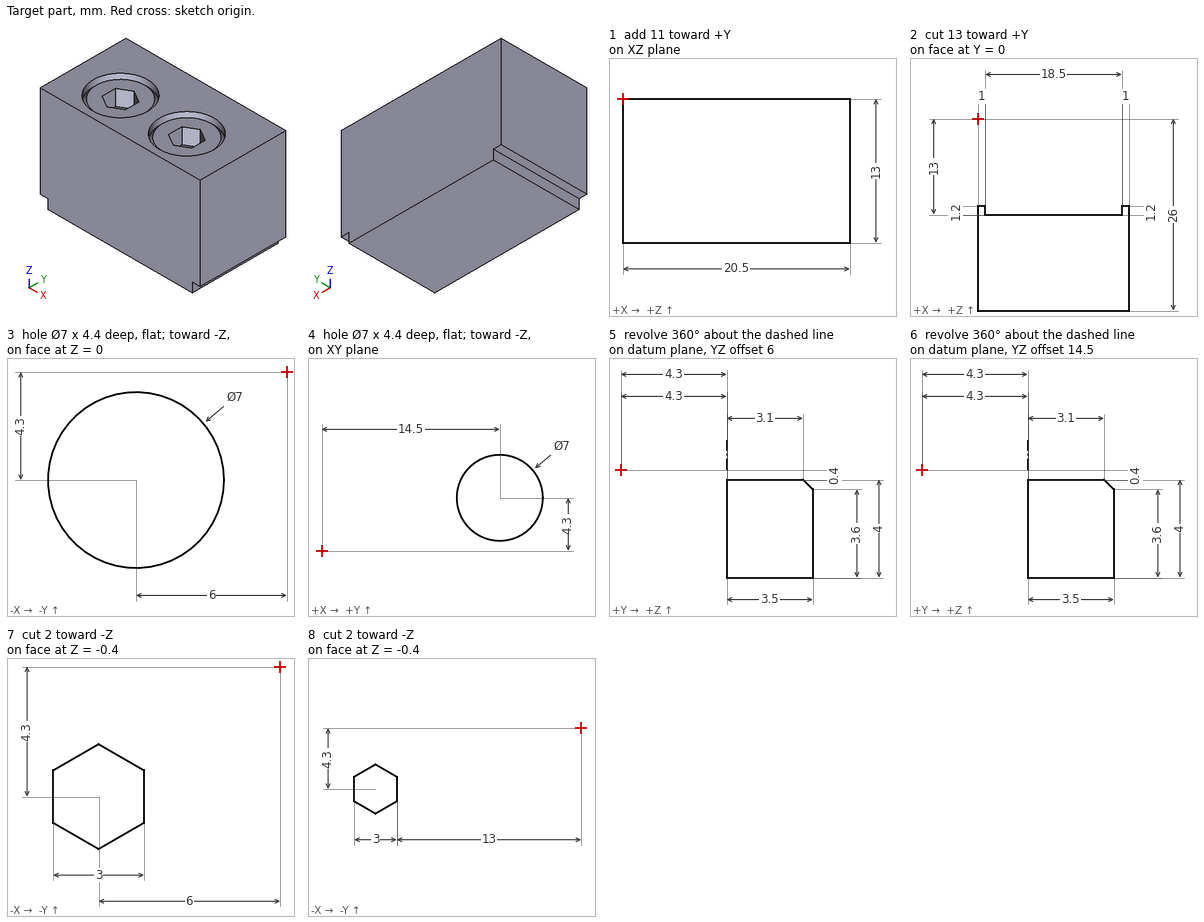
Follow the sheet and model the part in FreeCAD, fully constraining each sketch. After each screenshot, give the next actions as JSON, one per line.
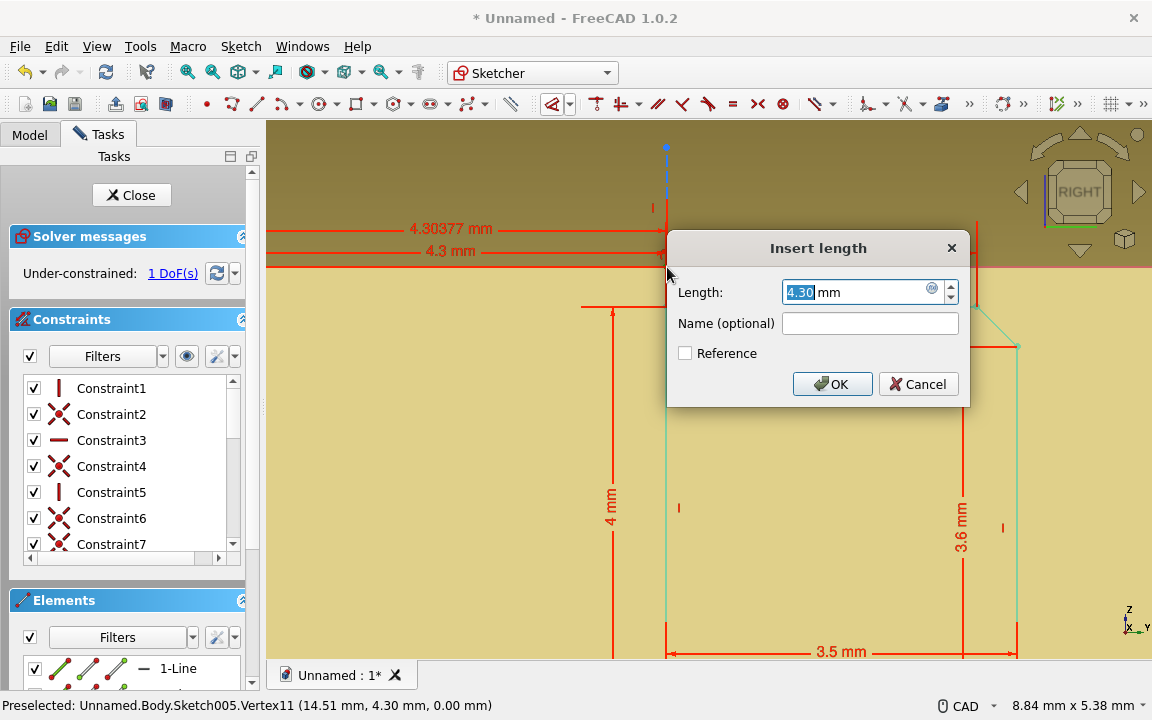
{"action": "type", "text": "4.3"}
{"action": "key", "text": "Return"}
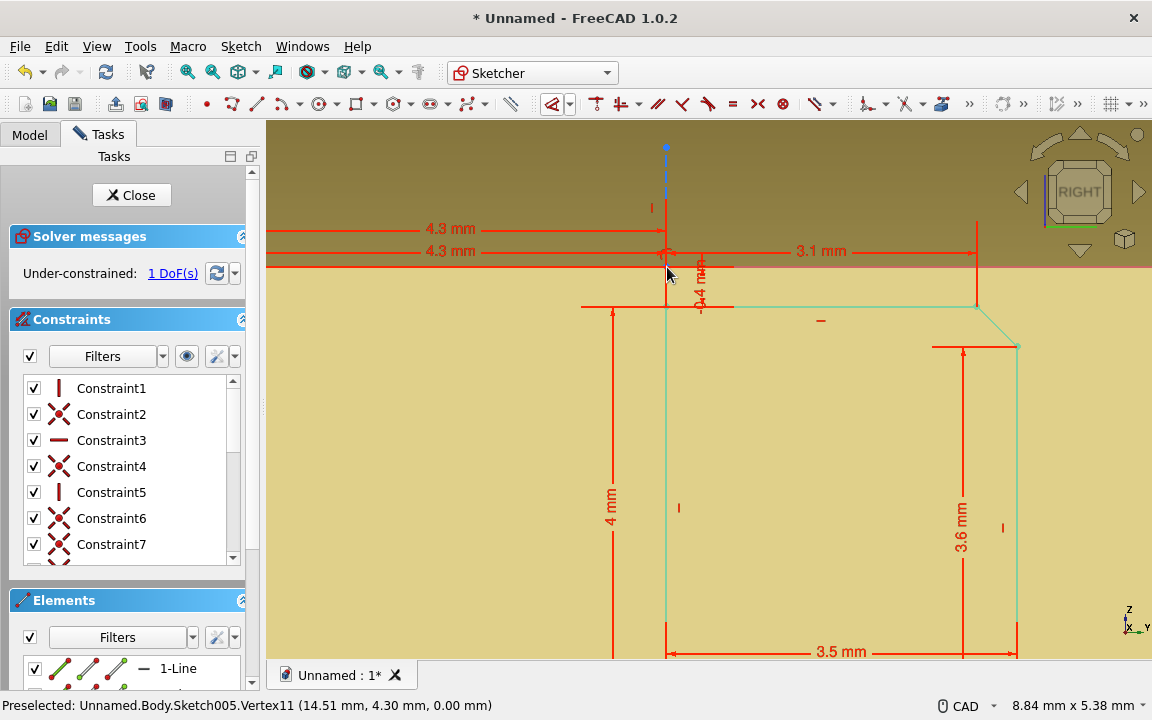
{"action": "left_click", "coordinate": [132, 195]}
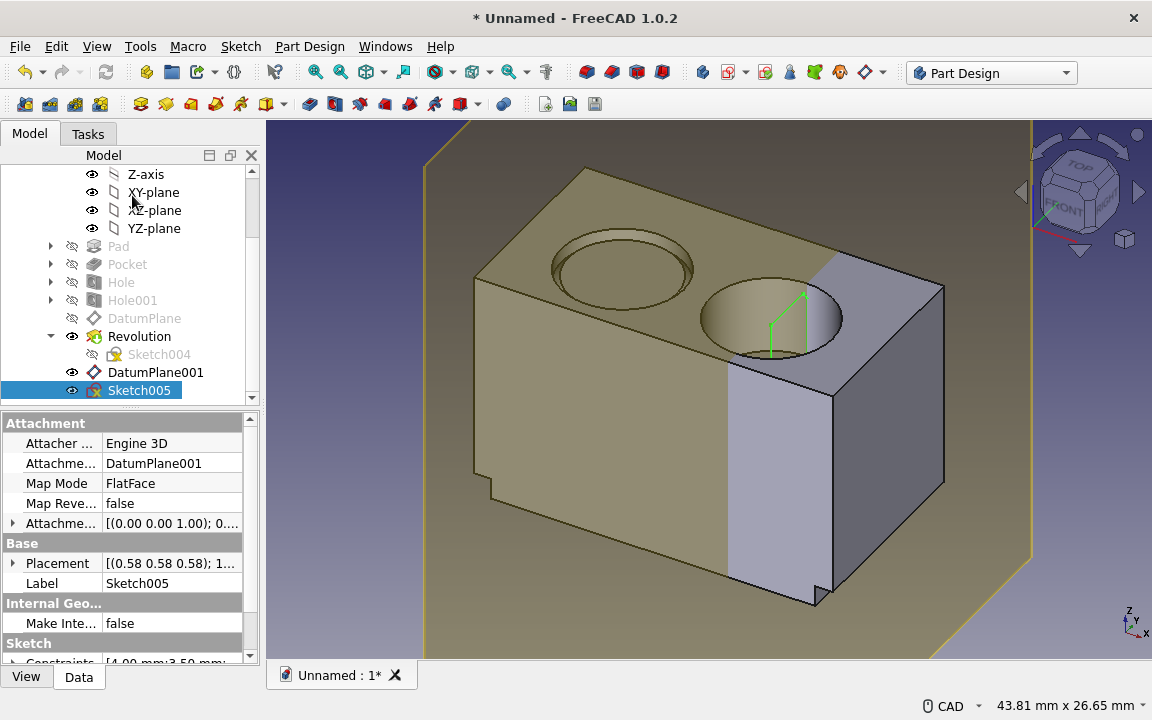
{"action": "left_click", "coordinate": [166, 104]}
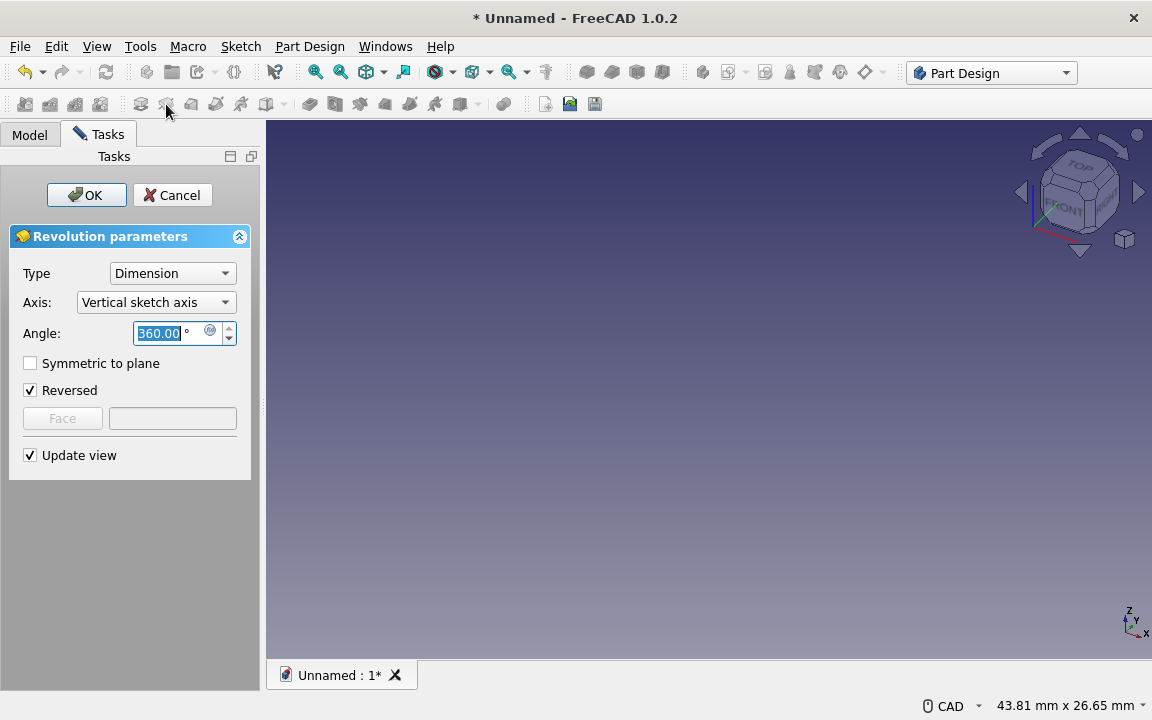
{"action": "left_click", "coordinate": [157, 302]}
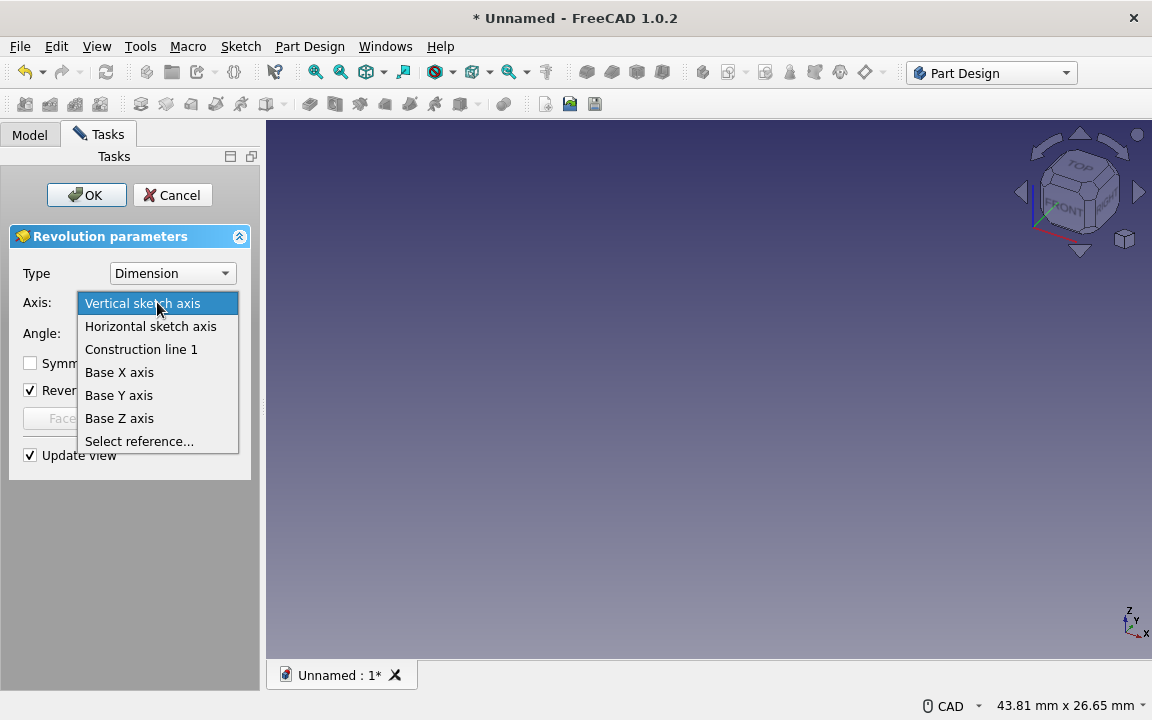
{"action": "left_click", "coordinate": [156, 350]}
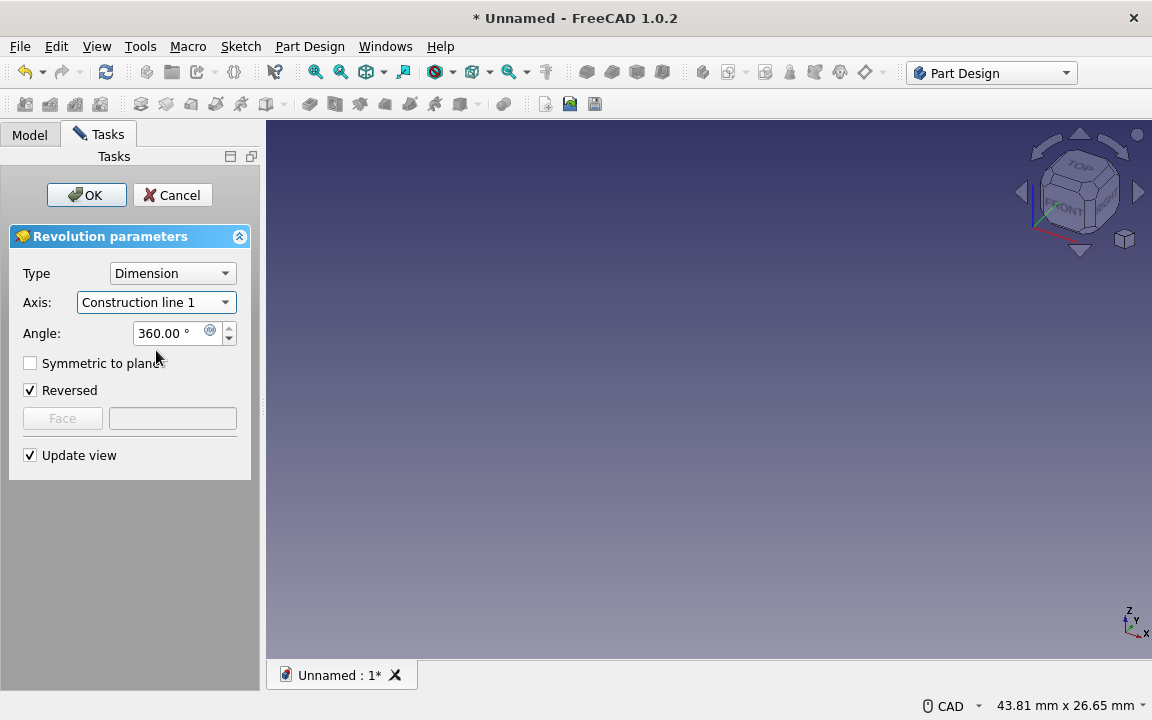
{"action": "left_click", "coordinate": [87, 195]}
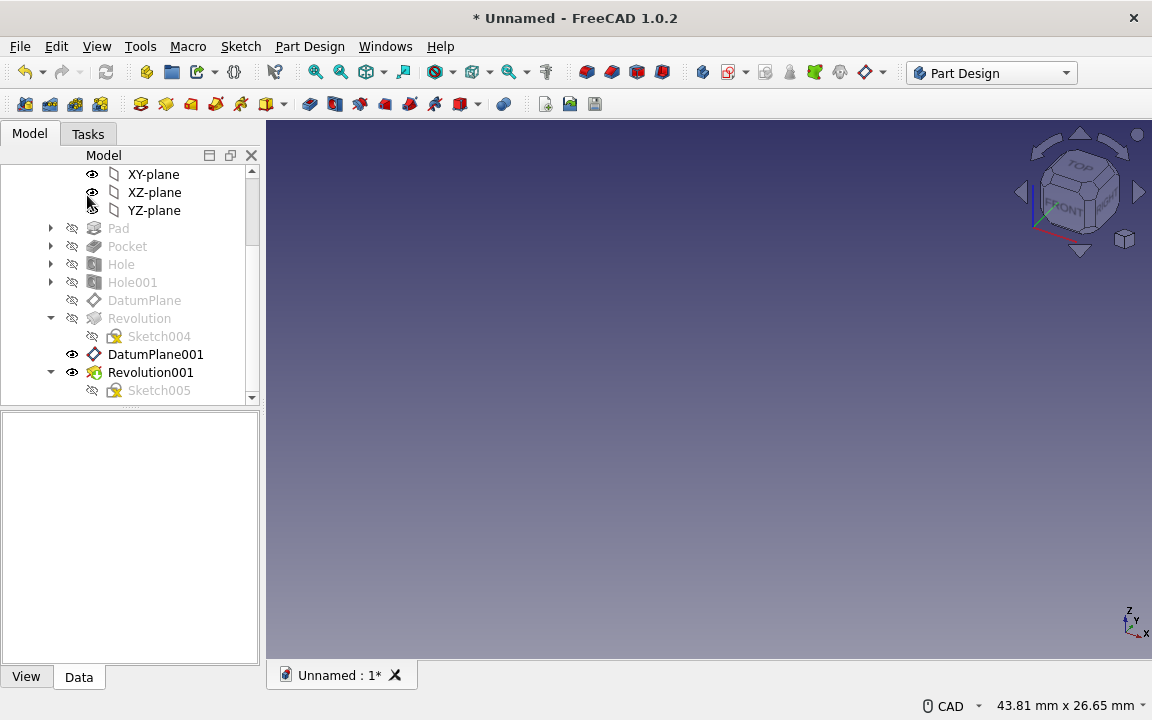
{"action": "left_click", "coordinate": [117, 354]}
{"action": "key", "text": "space"}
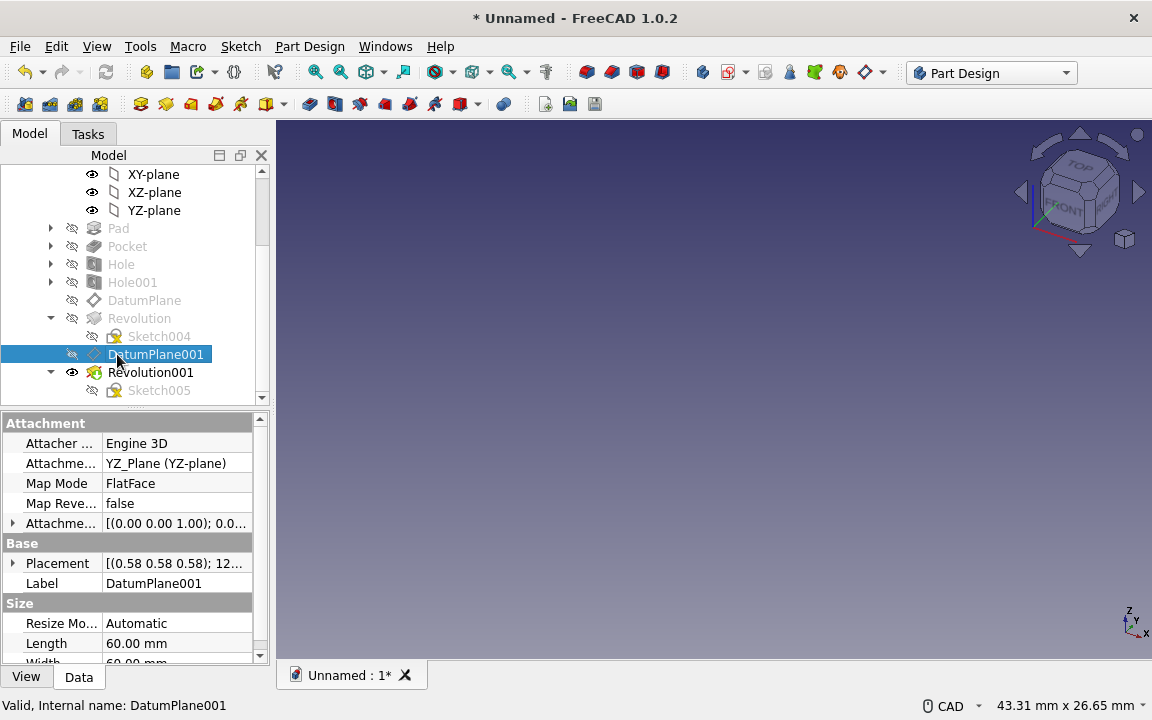
{"action": "left_click", "coordinate": [316, 72]}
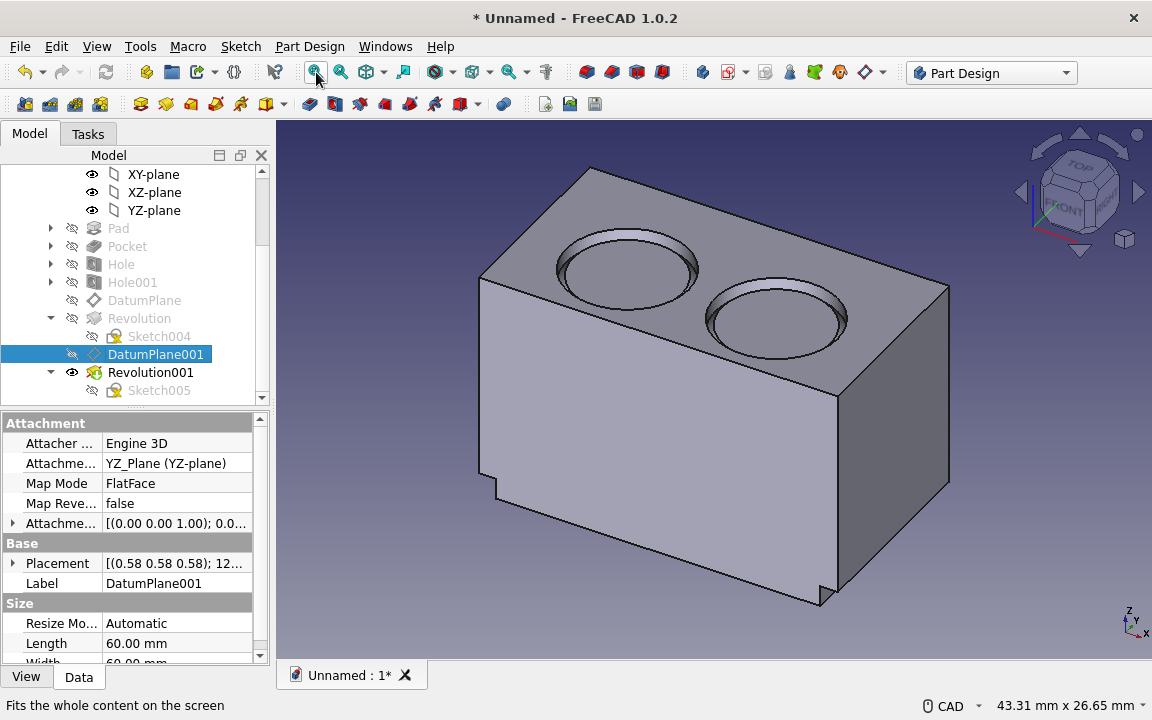
{"action": "left_click", "coordinate": [627, 275]}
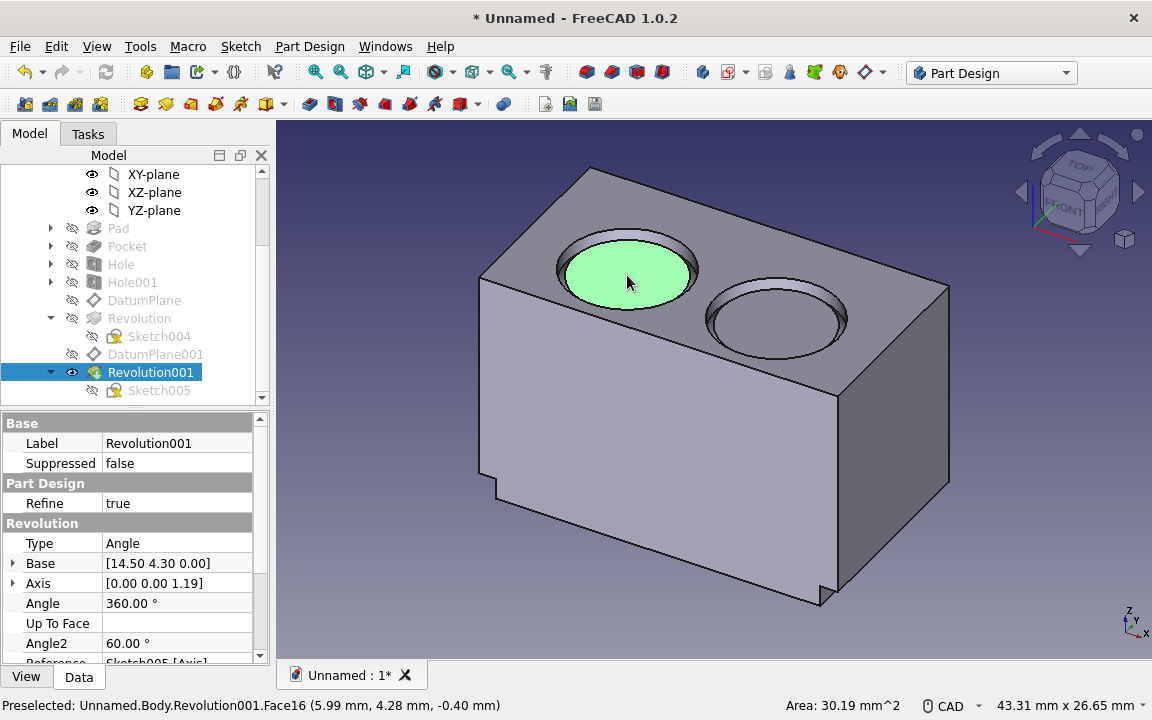
{"action": "left_click", "coordinate": [728, 72]}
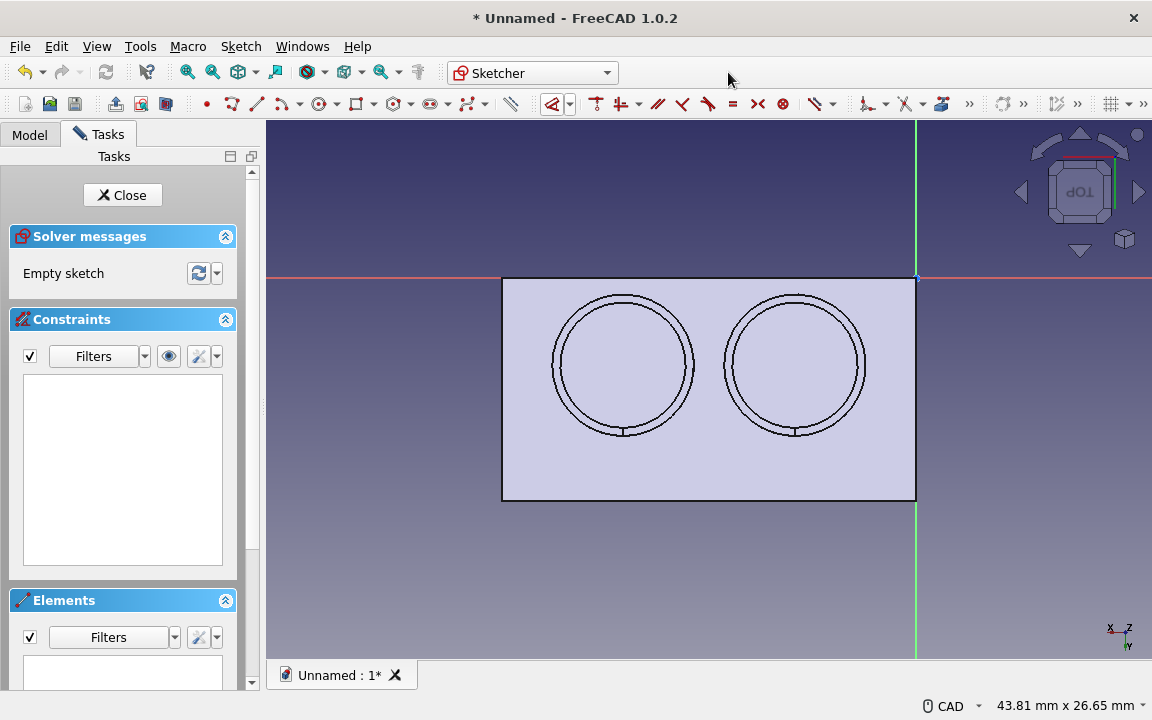
{"action": "scroll", "coordinate": [957, 310], "scroll_direction": "up", "scroll_amount": 5}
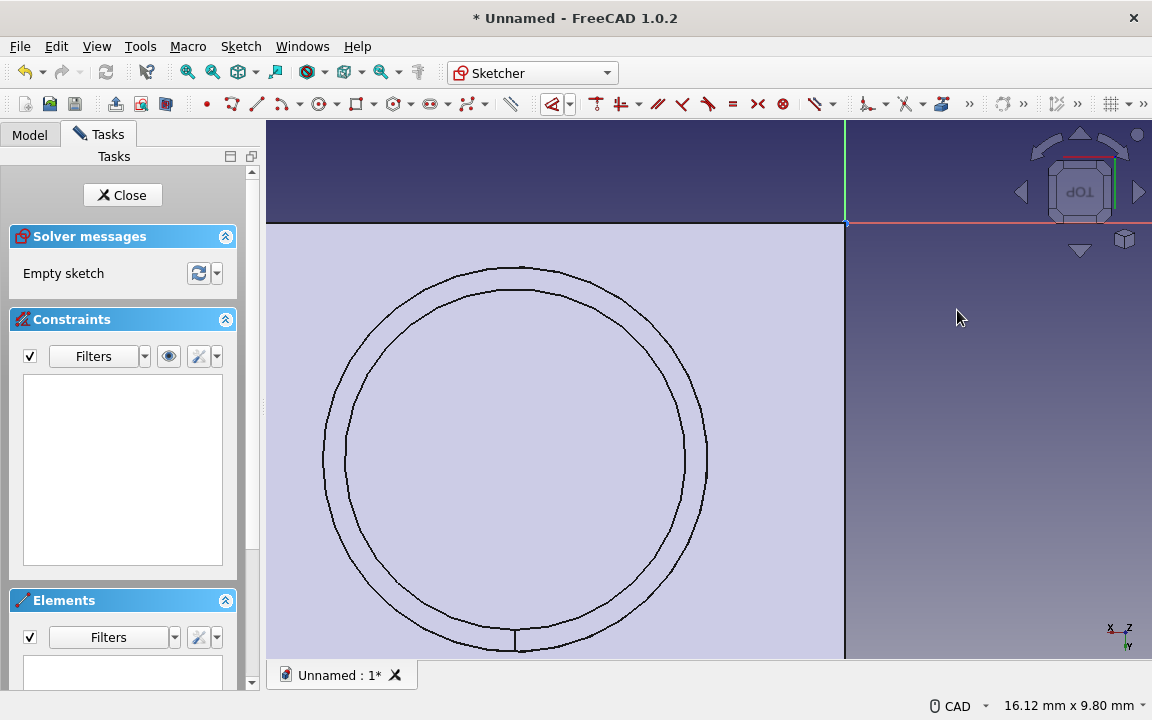
{"action": "left_click", "coordinate": [392, 104]}